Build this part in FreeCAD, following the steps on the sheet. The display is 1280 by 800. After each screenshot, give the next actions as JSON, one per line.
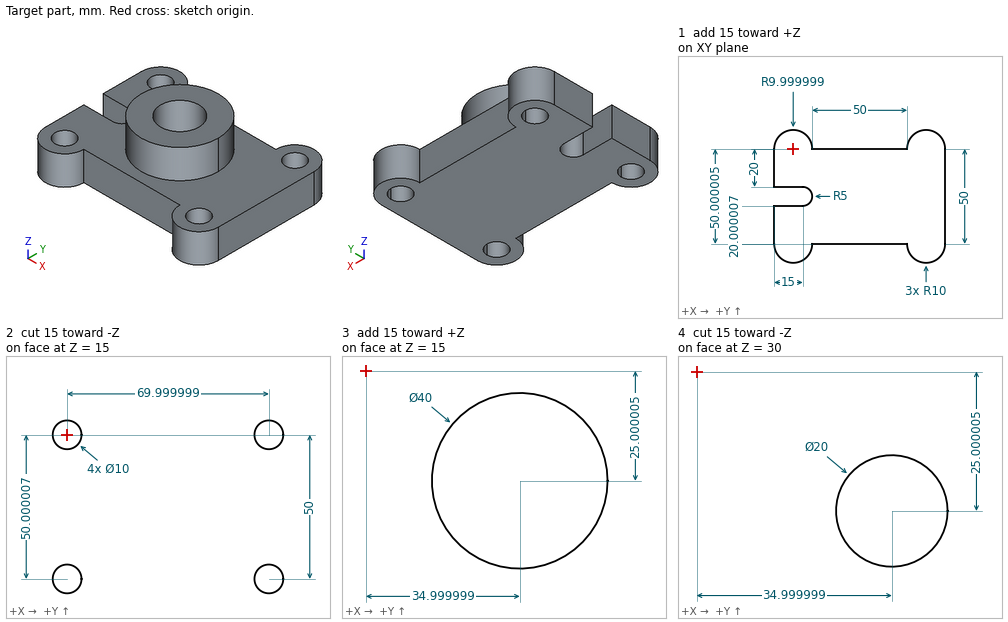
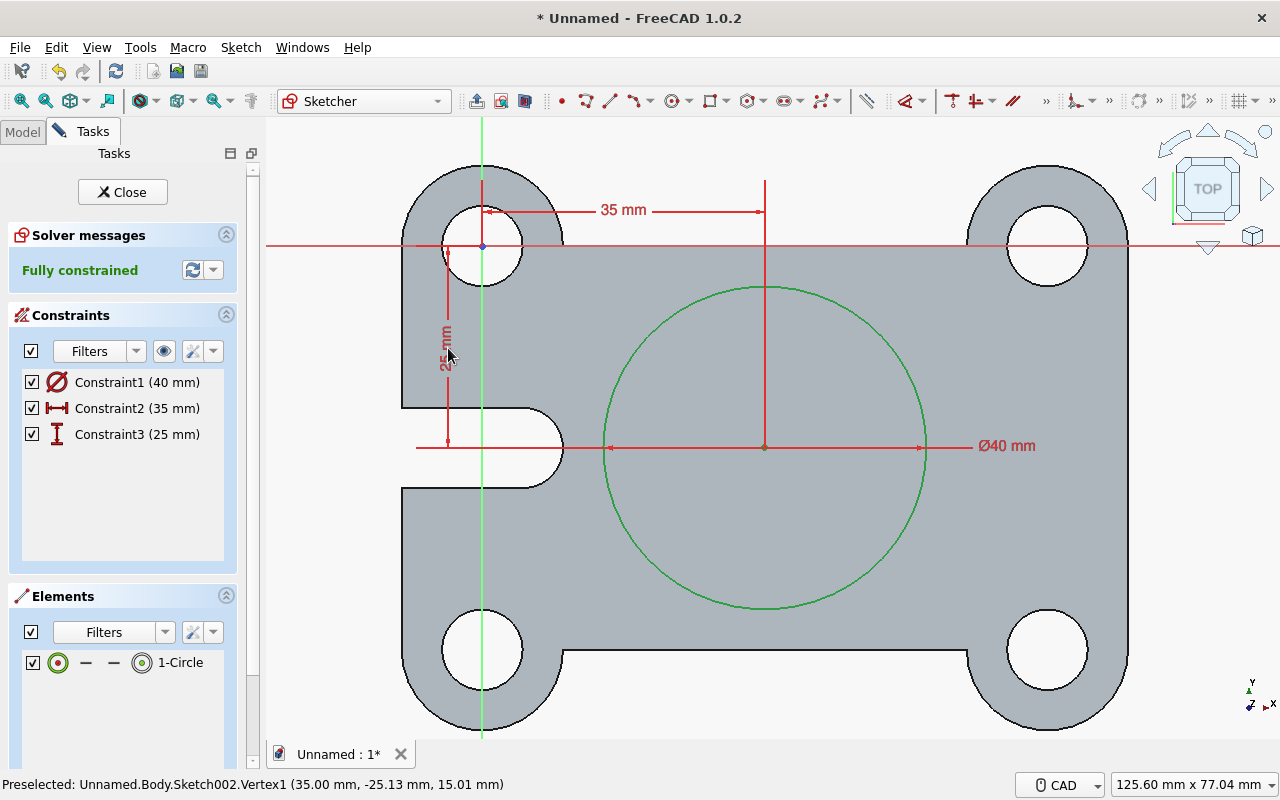
{"action": "left_click", "coordinate": [123, 192]}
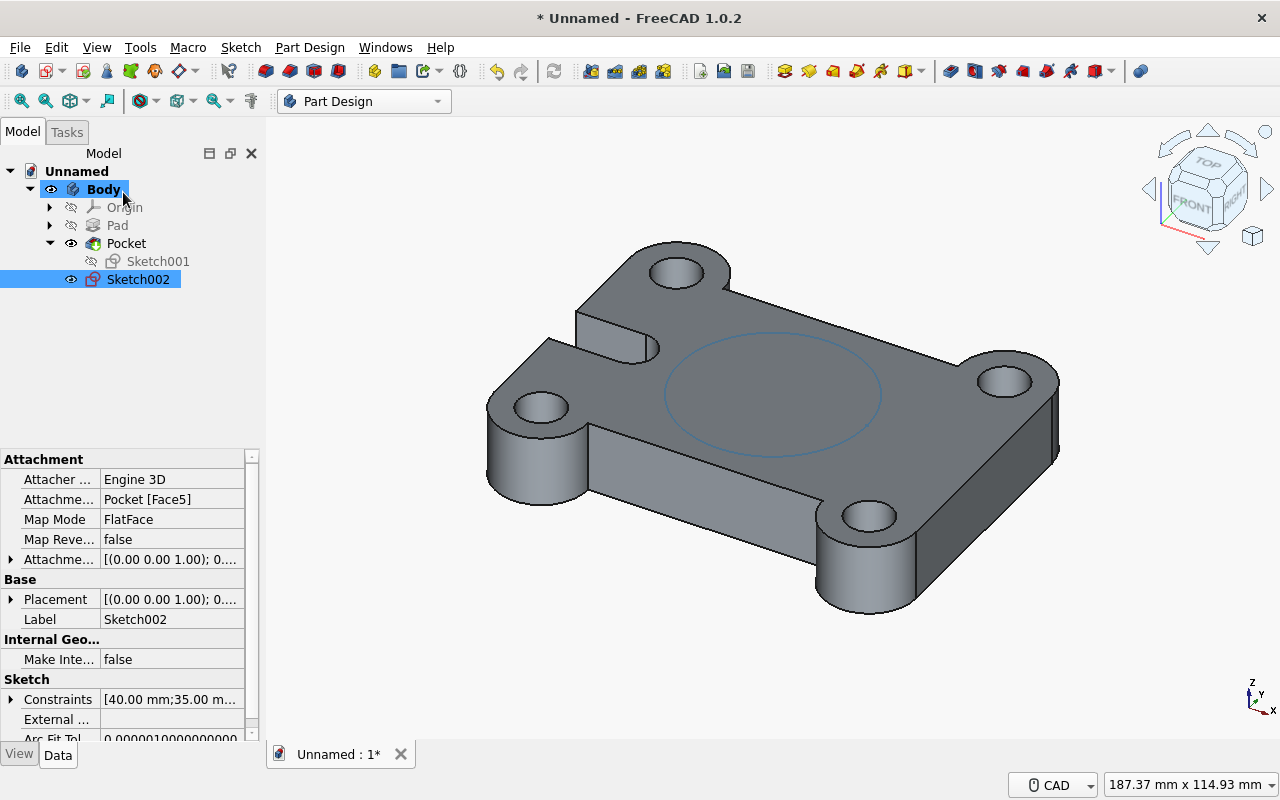
{"action": "left_click", "coordinate": [786, 72]}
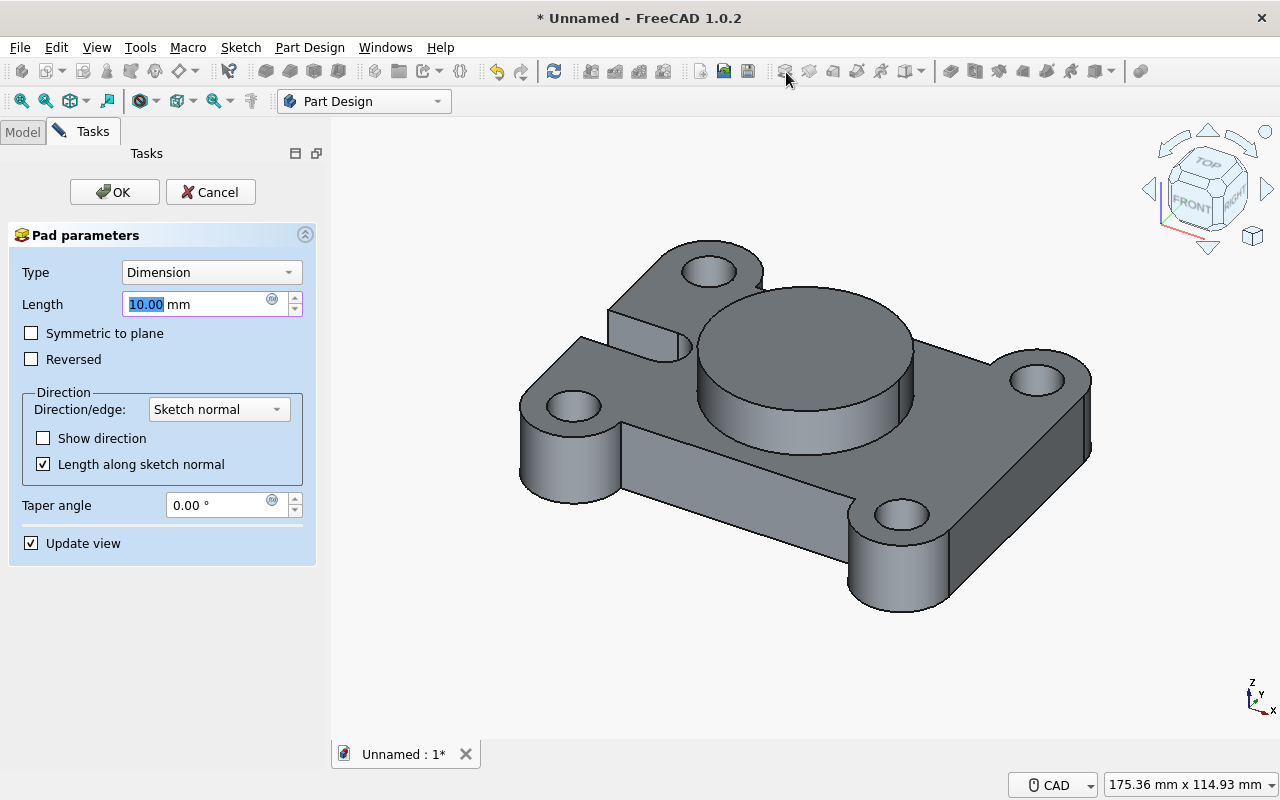
{"action": "type", "text": "15"}
{"action": "key", "text": "Tab"}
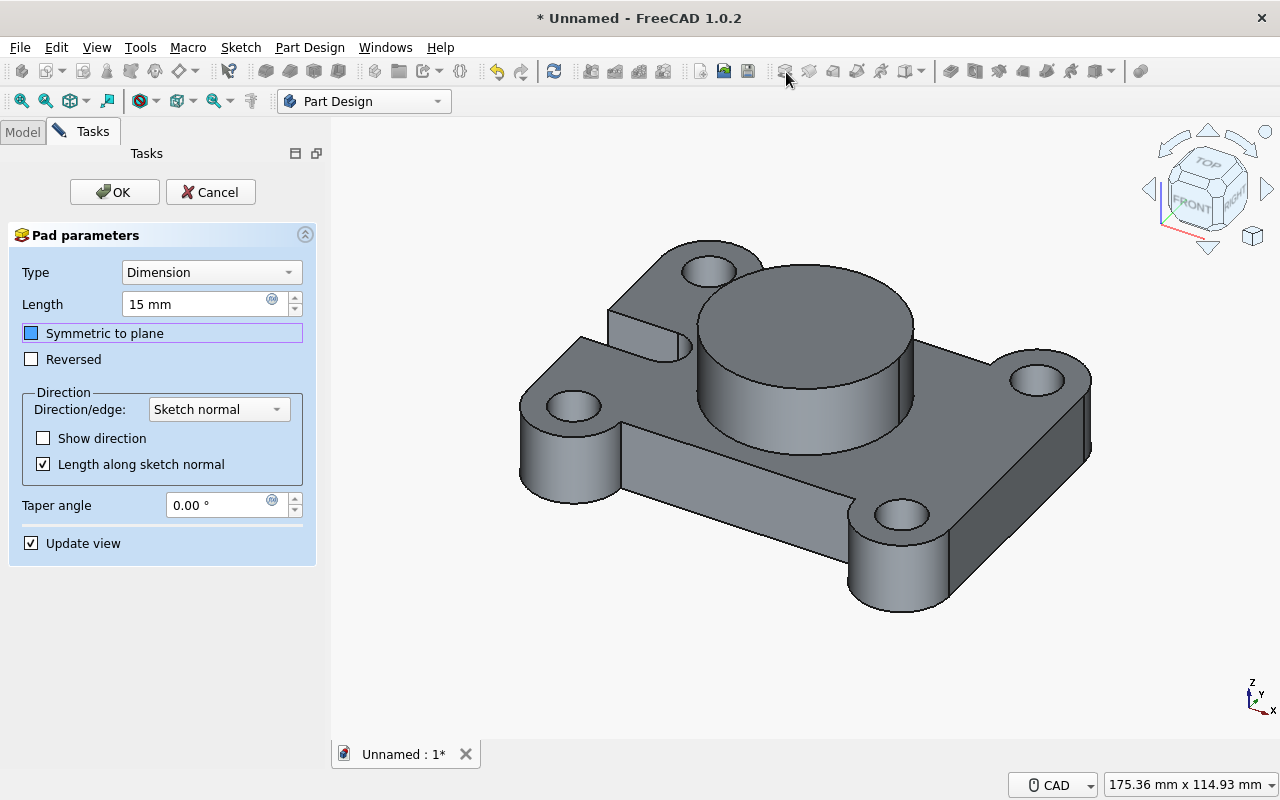
{"action": "left_click", "coordinate": [115, 192]}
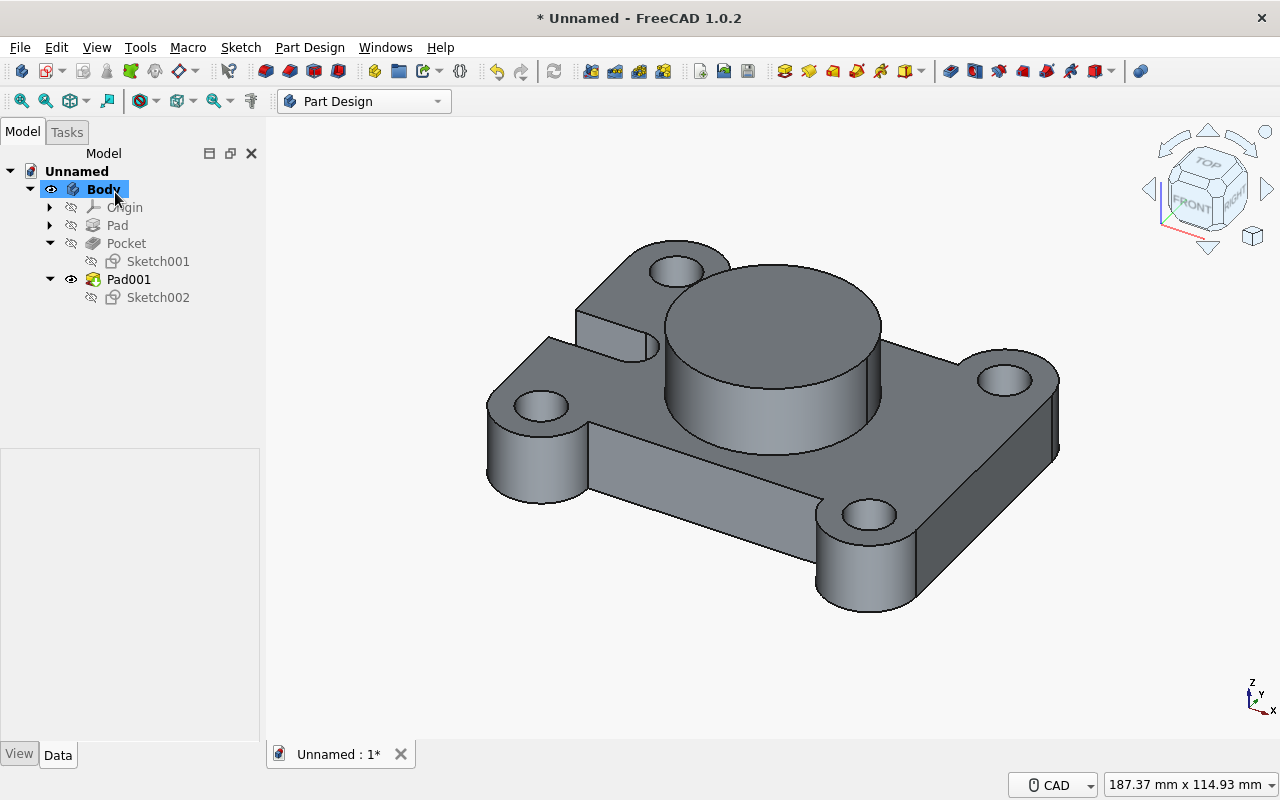
{"action": "left_click", "coordinate": [773, 326]}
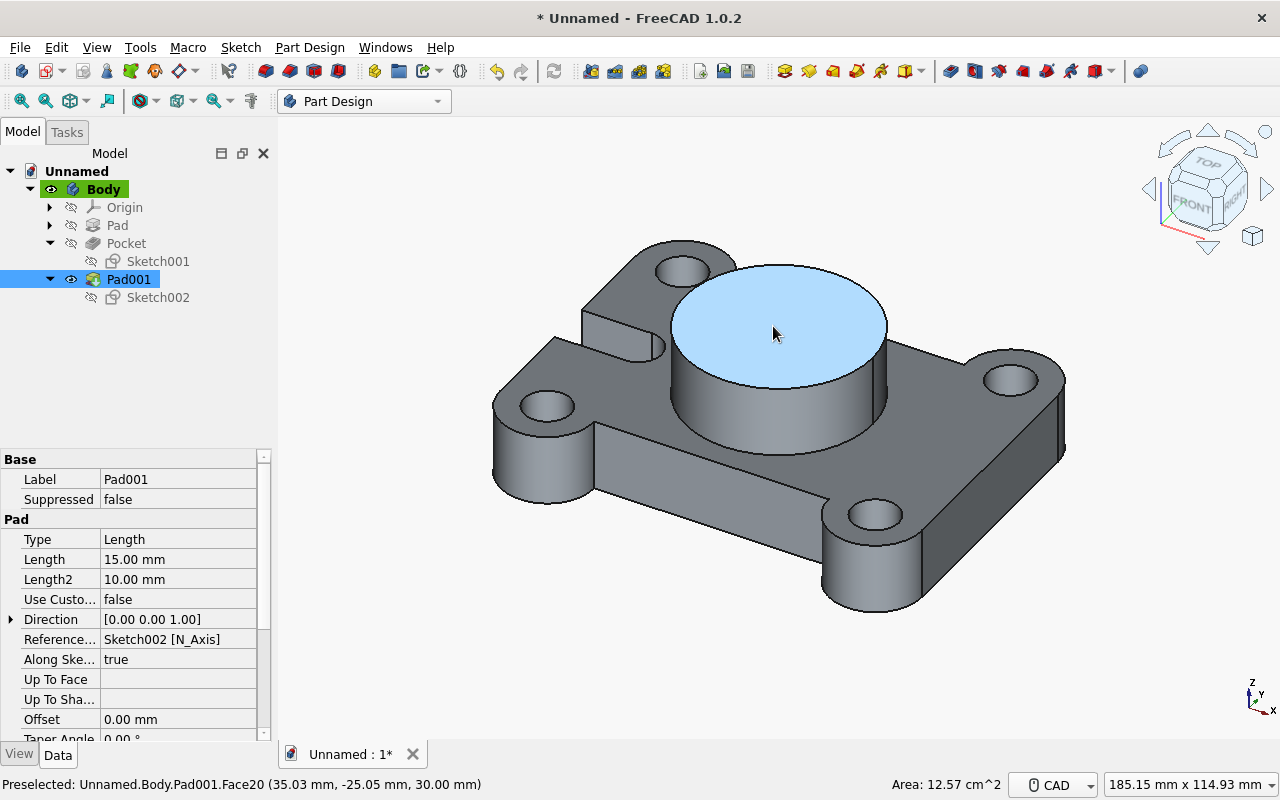
{"action": "left_click", "coordinate": [46, 72]}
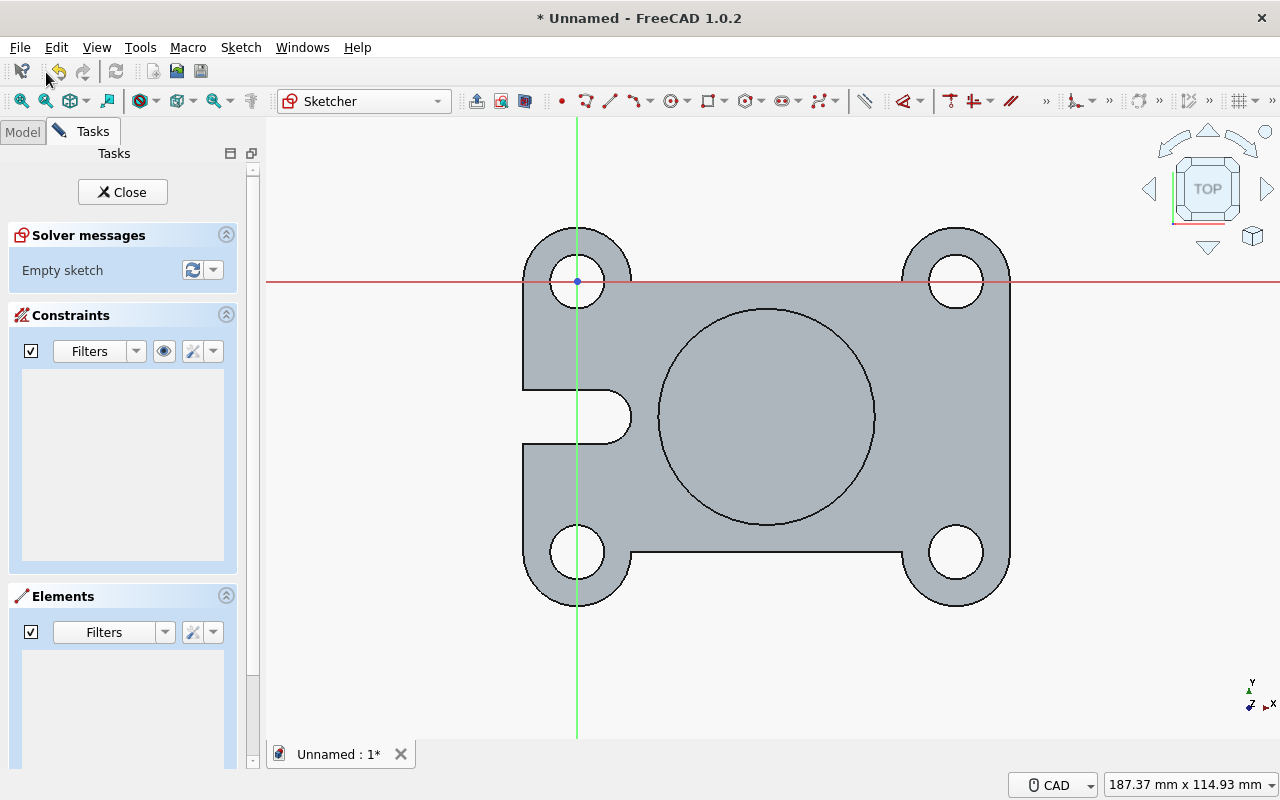
{"action": "scroll", "coordinate": [694, 334], "scroll_direction": "up", "scroll_amount": 4}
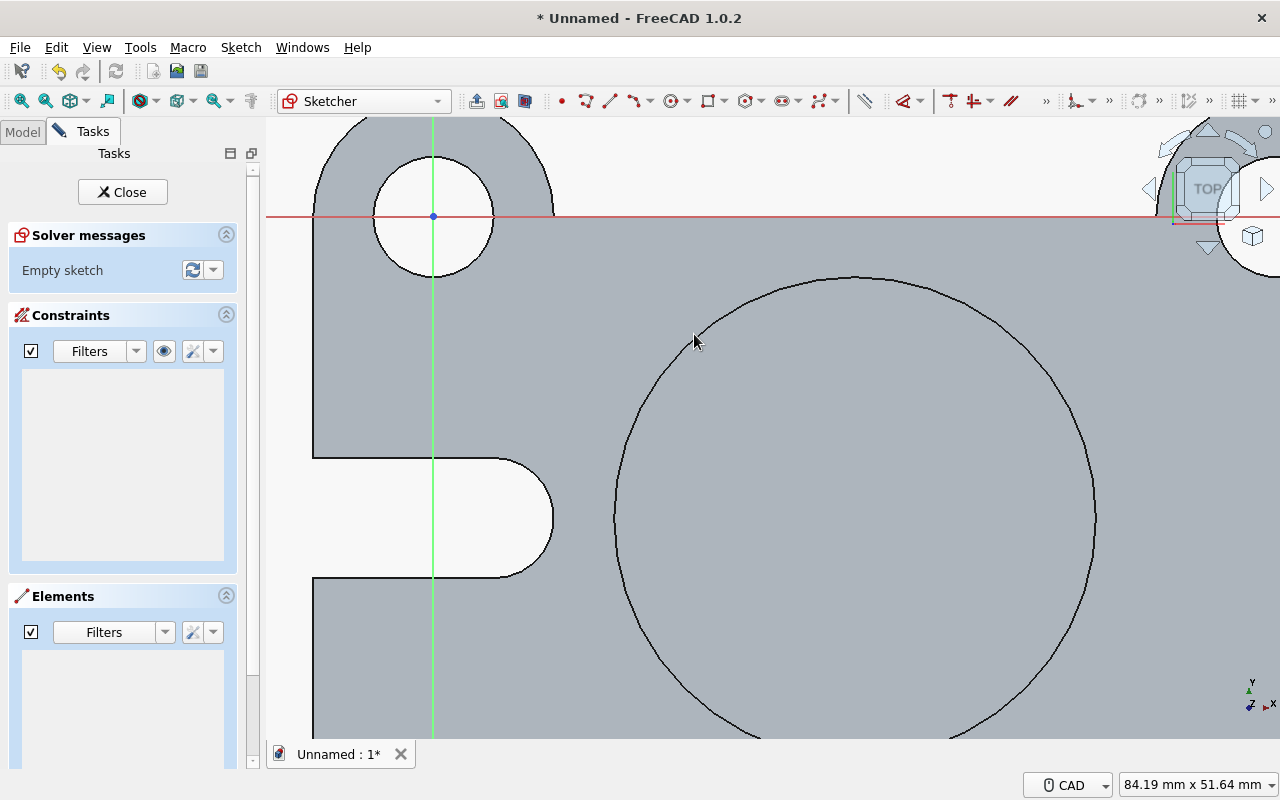
{"action": "left_click", "coordinate": [672, 102]}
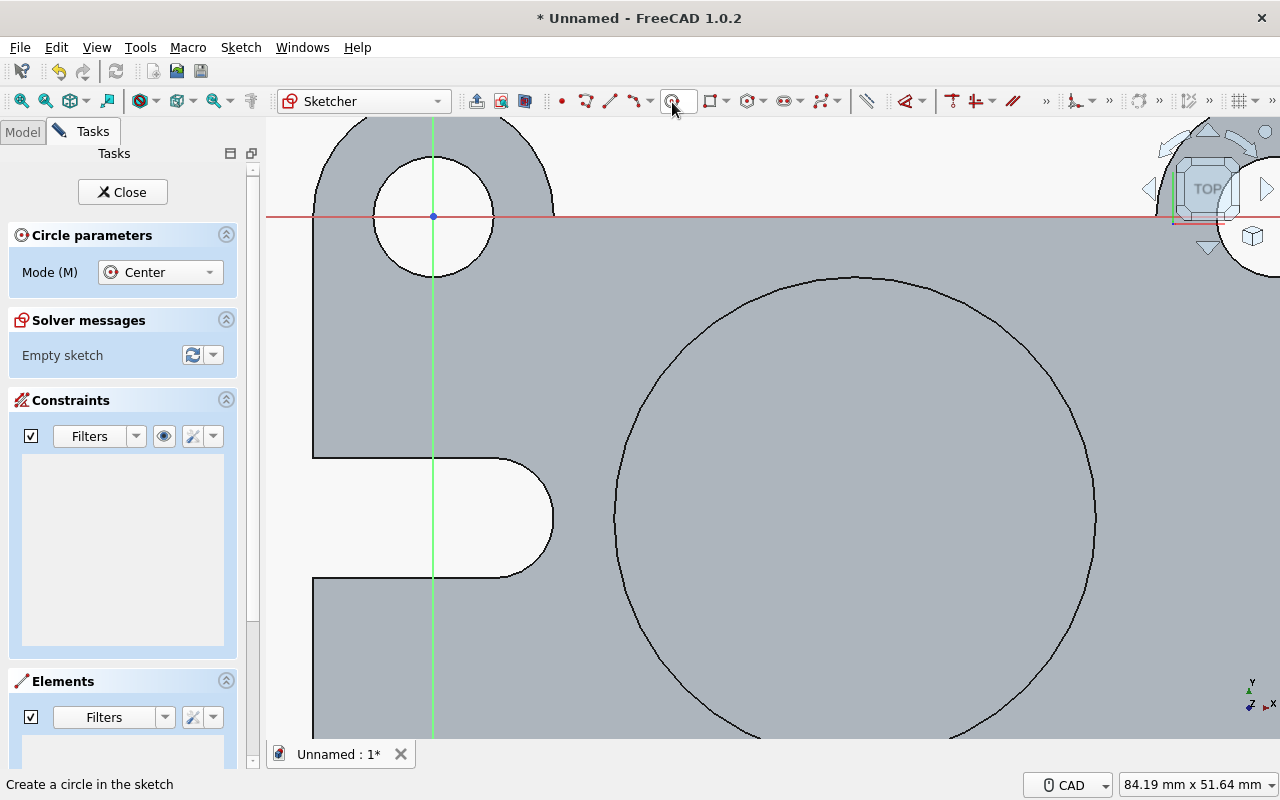
{"action": "left_click", "coordinate": [855, 518]}
{"action": "mouse_move", "coordinate": [940, 433]}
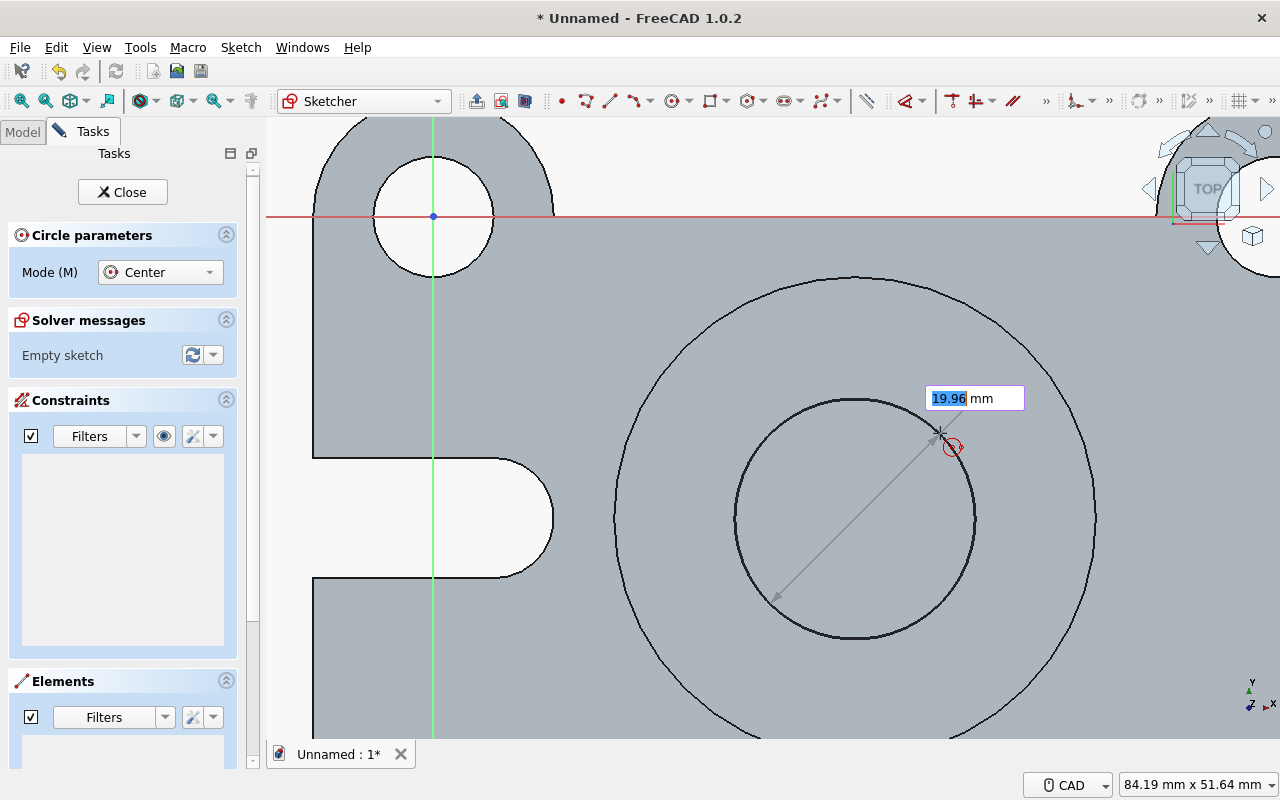
{"action": "type", "text": "20"}
{"action": "key", "text": "Return"}
{"action": "key", "text": "Escape"}